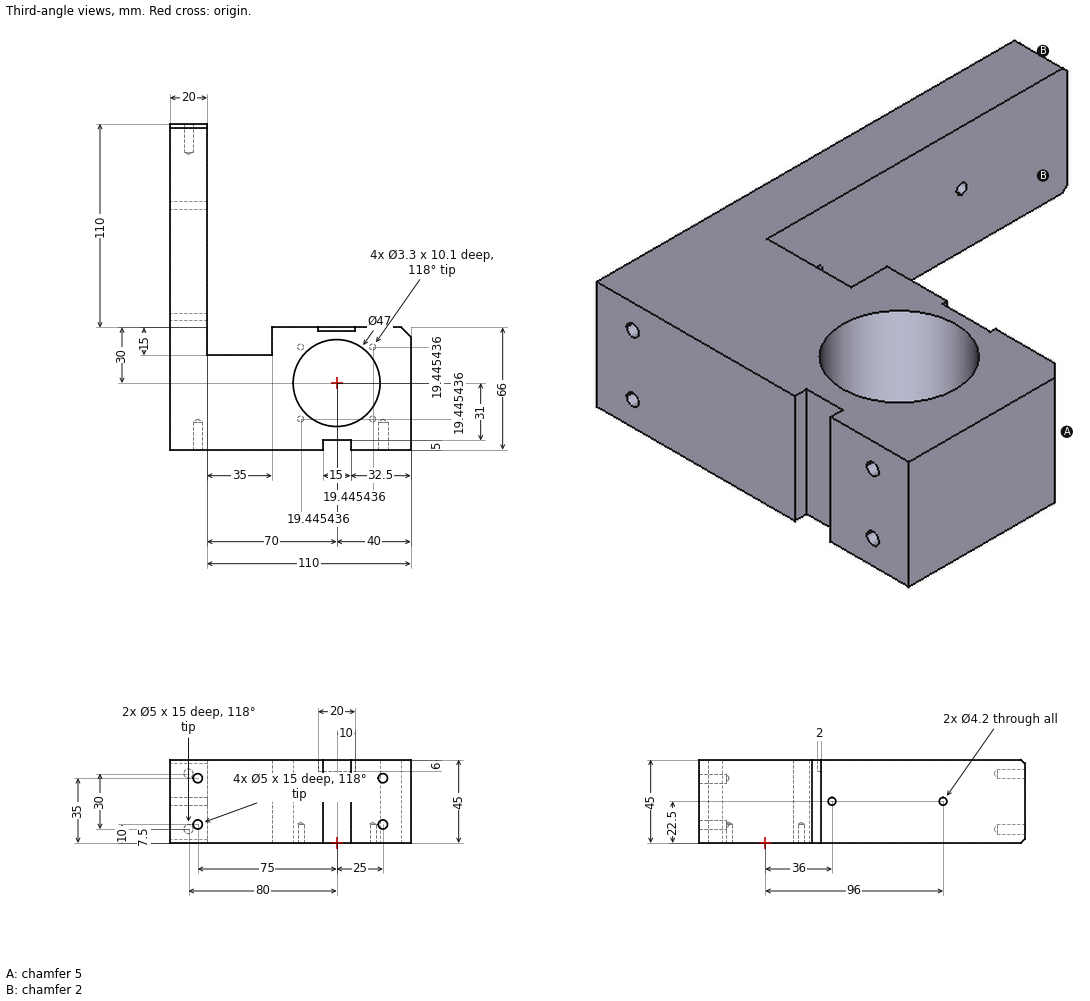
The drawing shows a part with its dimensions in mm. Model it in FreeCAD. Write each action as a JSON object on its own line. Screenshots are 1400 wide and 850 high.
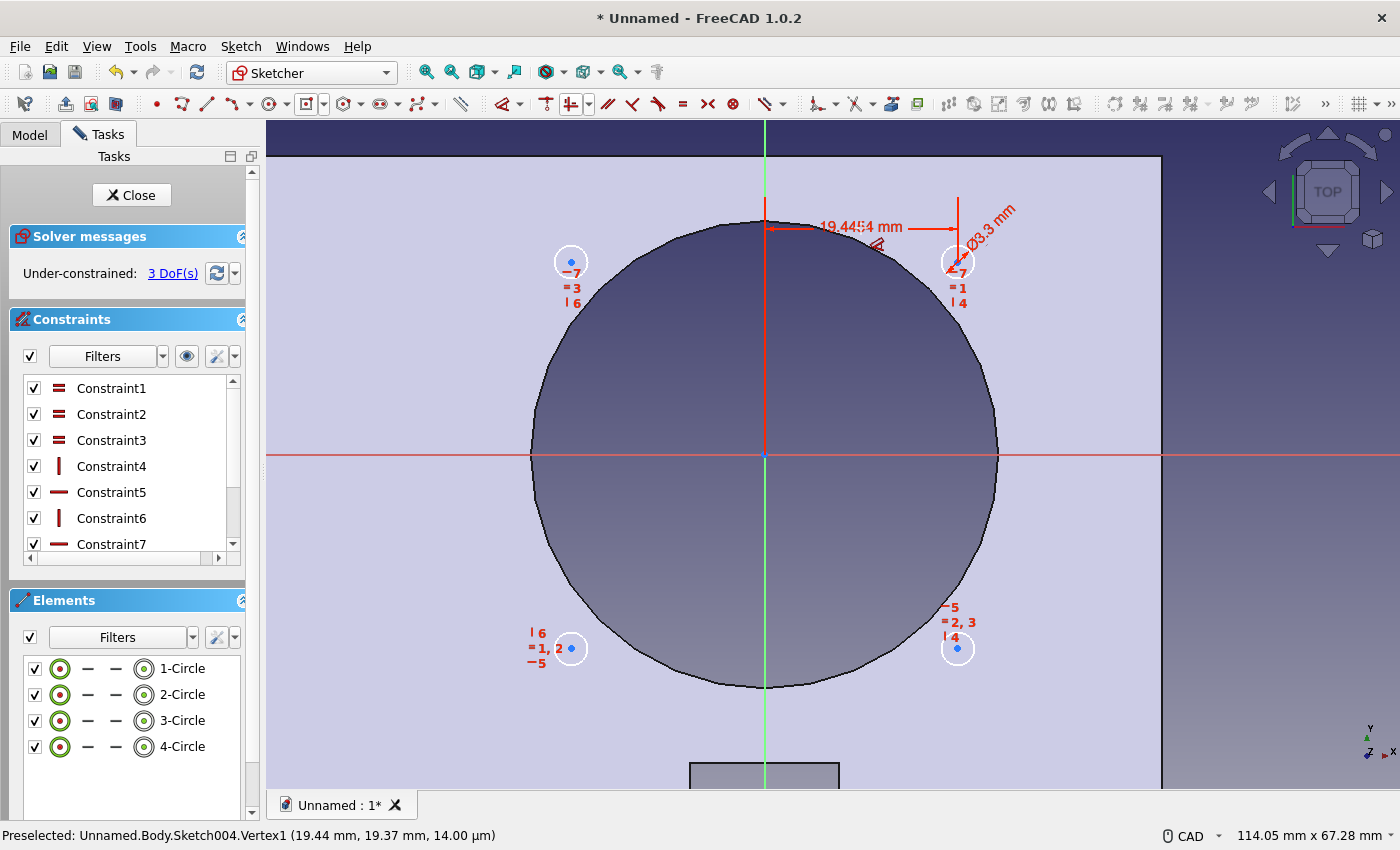
{"action": "left_click", "coordinate": [958, 262]}
{"action": "left_click", "coordinate": [992, 358]}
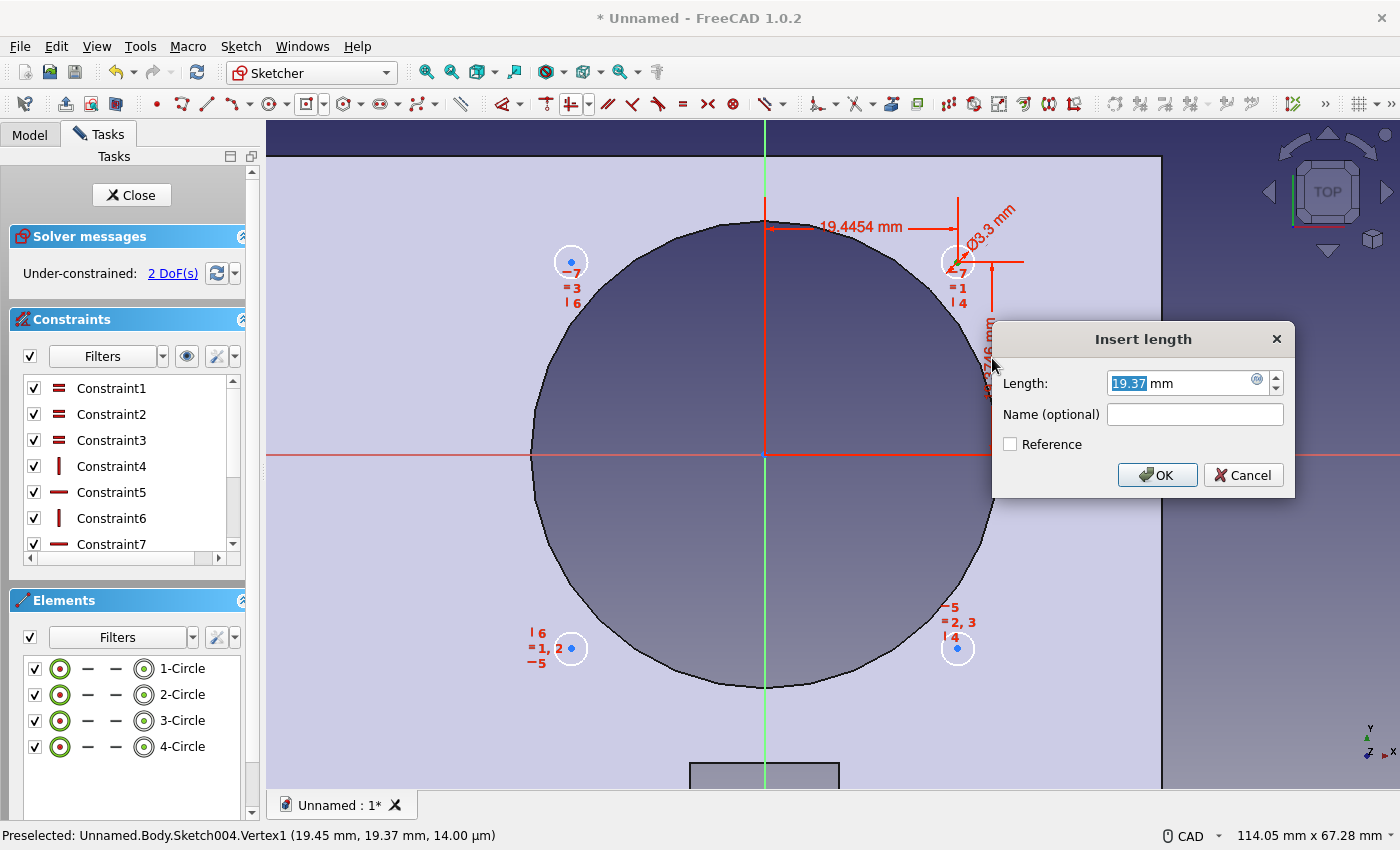
{"action": "type", "text": "19.445436"}
{"action": "key", "text": "Return"}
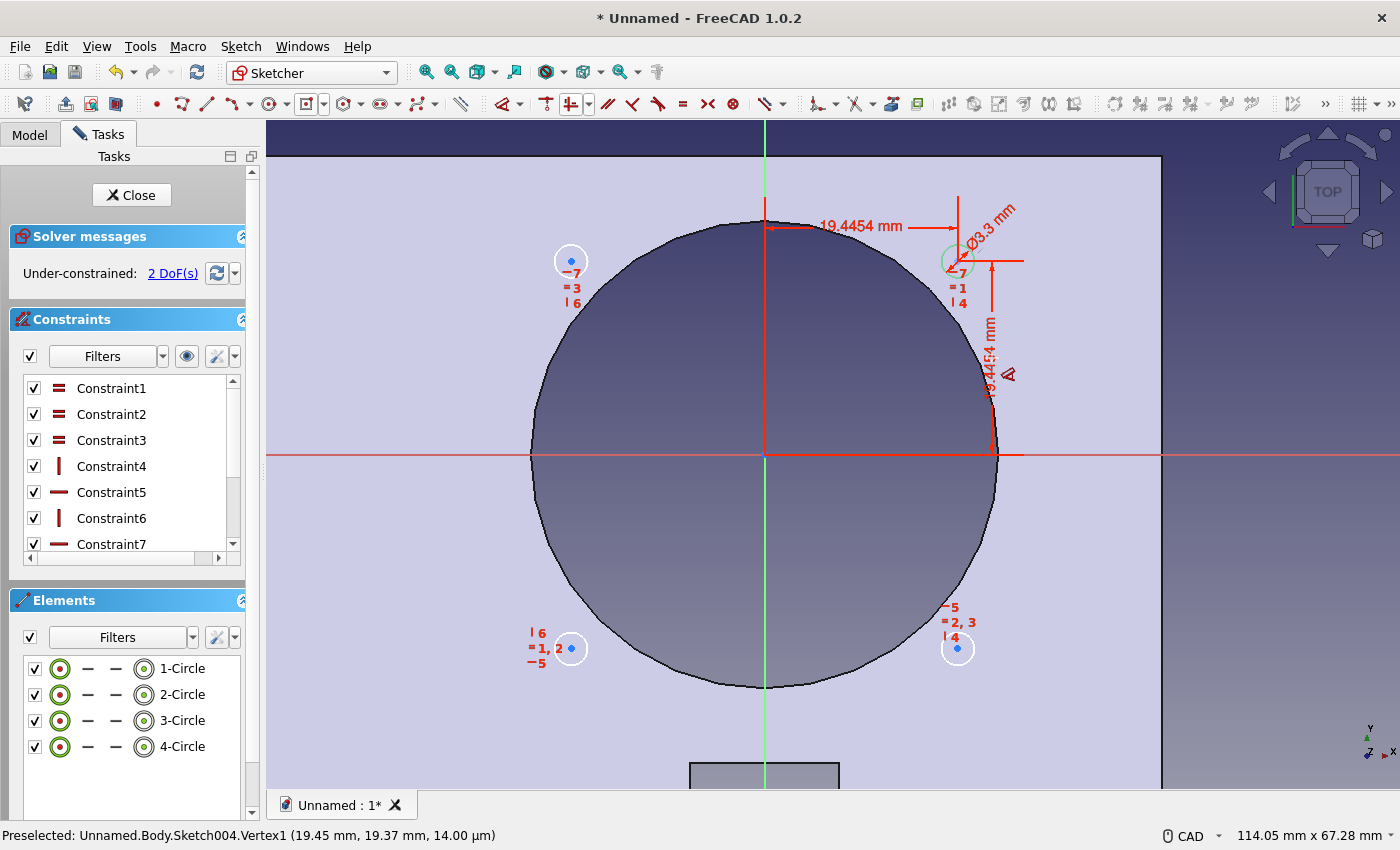
{"action": "left_click", "coordinate": [571, 649]}
{"action": "left_click", "coordinate": [668, 683]}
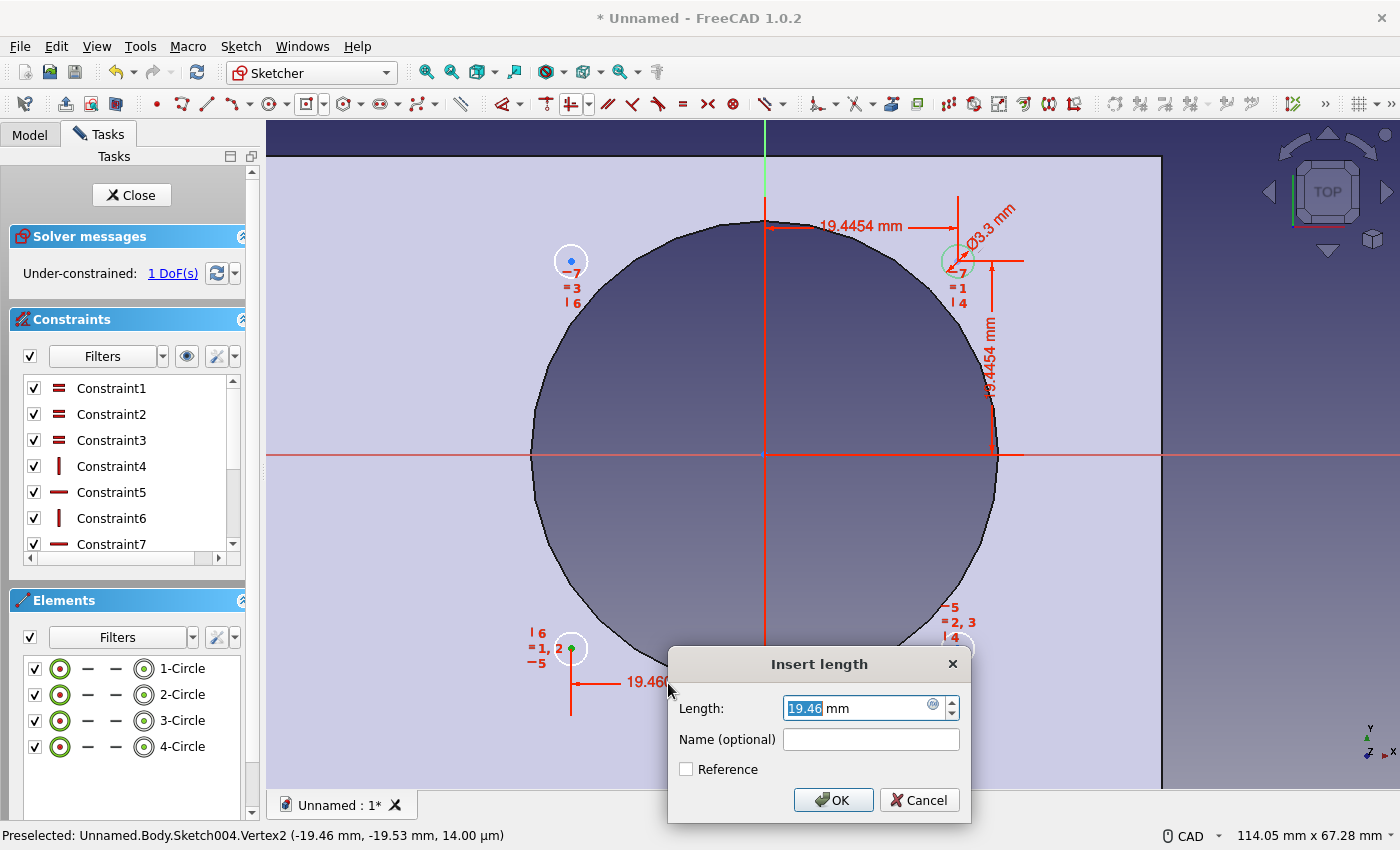
{"action": "type", "text": "19.445436"}
{"action": "key", "text": "Return"}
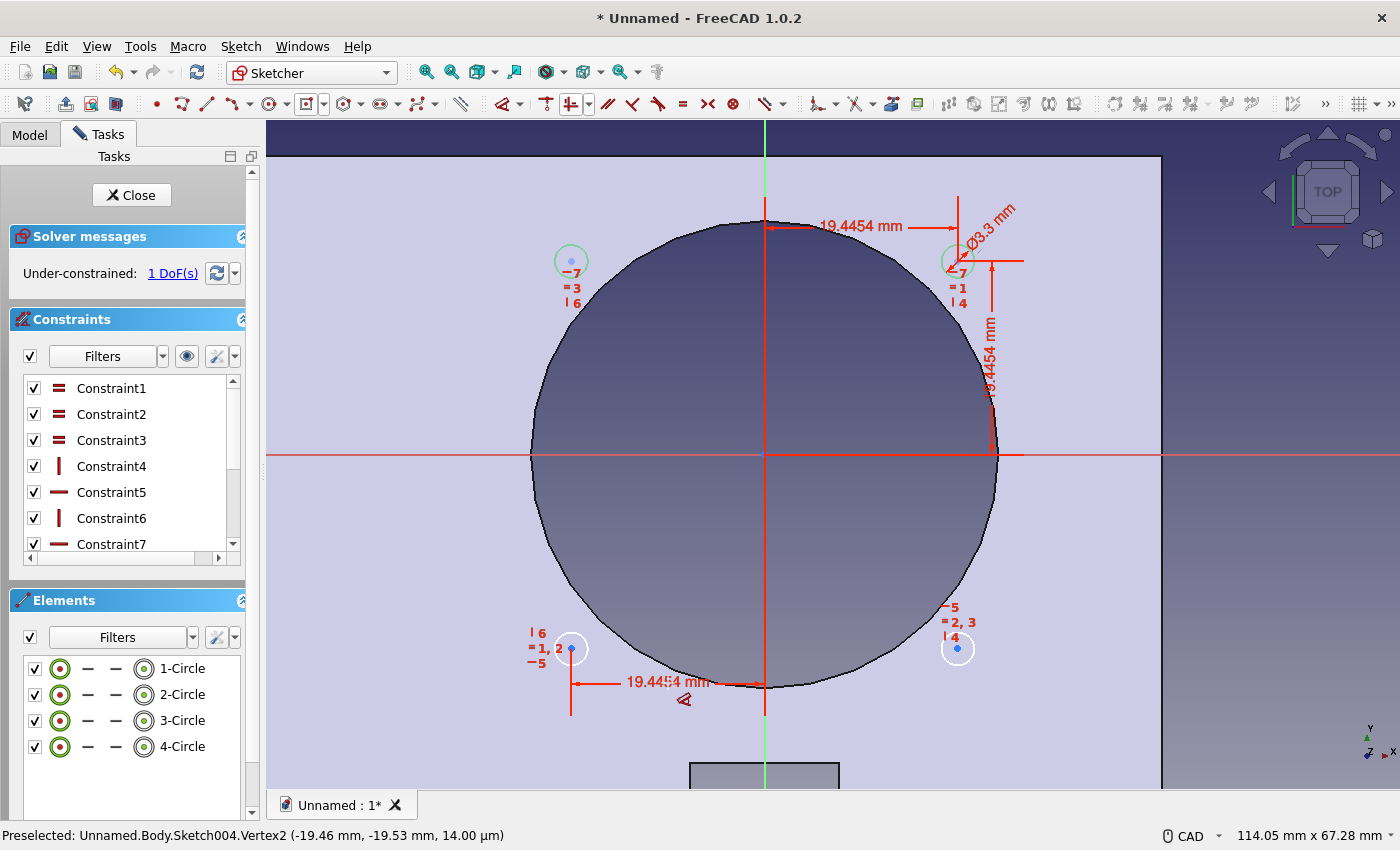
{"action": "left_click", "coordinate": [571, 649]}
{"action": "left_click", "coordinate": [537, 552]}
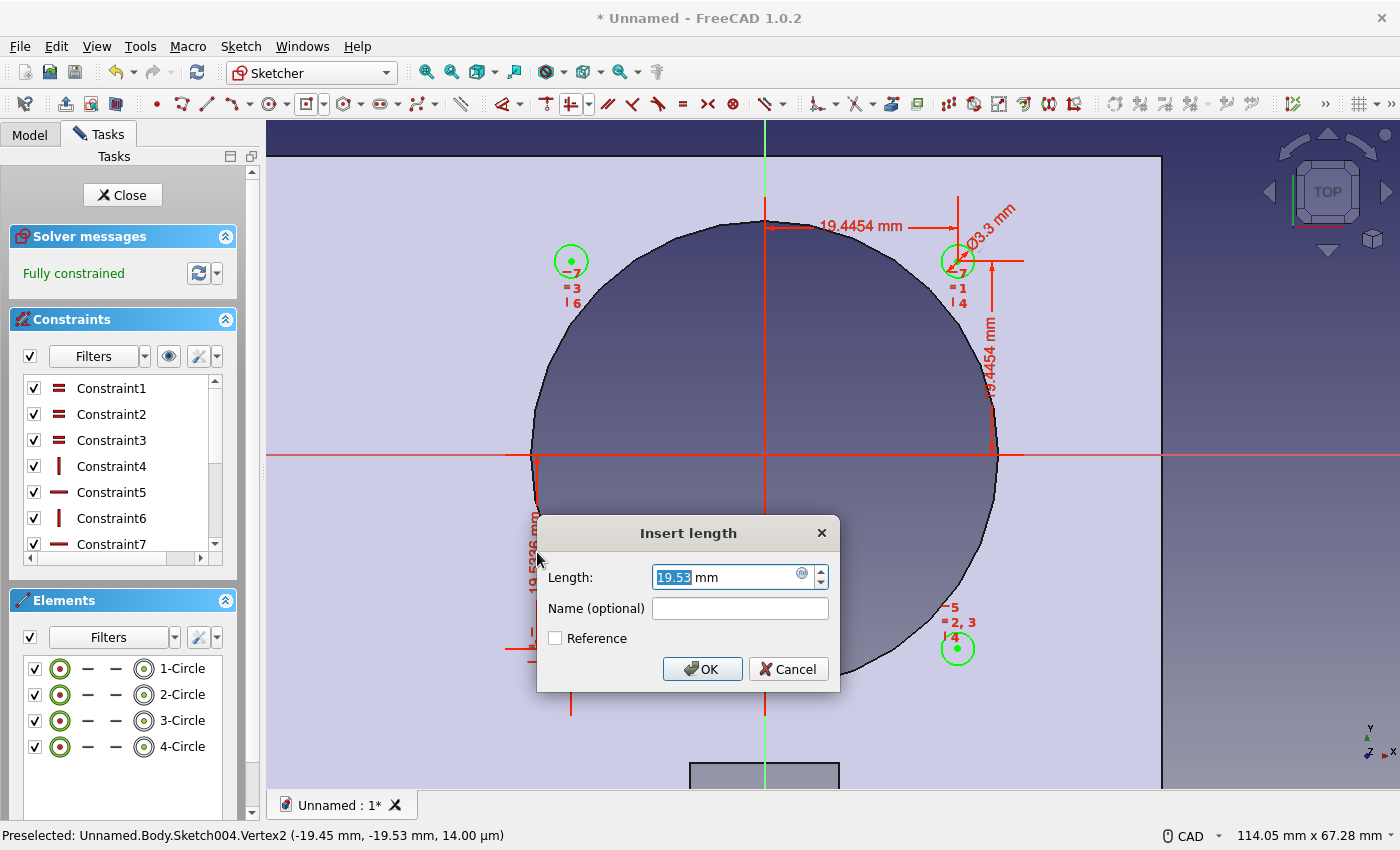
{"action": "type", "text": "19.445436"}
{"action": "key", "text": "Return"}
{"action": "key", "text": "Escape"}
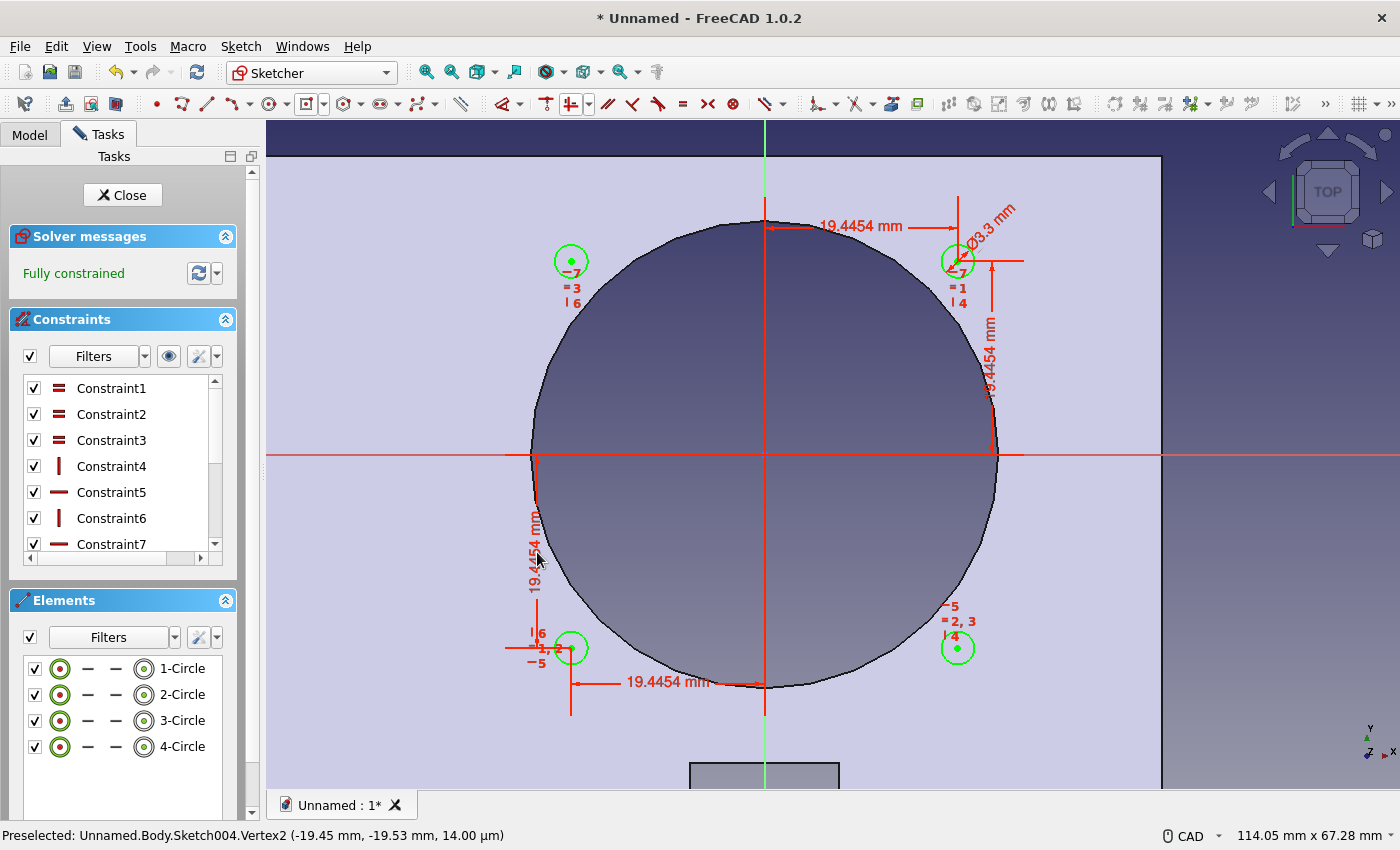
{"action": "left_click", "coordinate": [123, 195]}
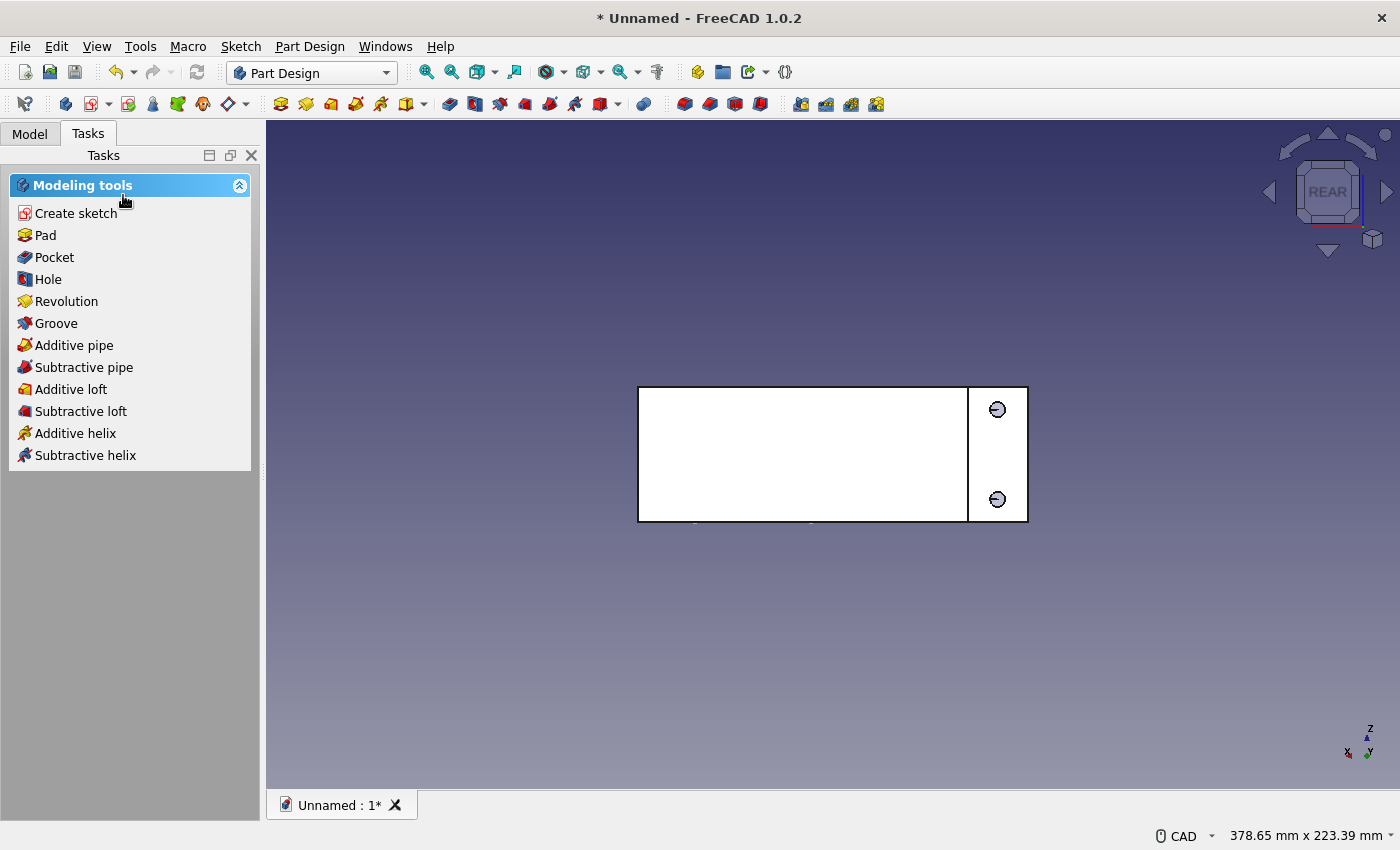
{"action": "left_click", "coordinate": [475, 104]}